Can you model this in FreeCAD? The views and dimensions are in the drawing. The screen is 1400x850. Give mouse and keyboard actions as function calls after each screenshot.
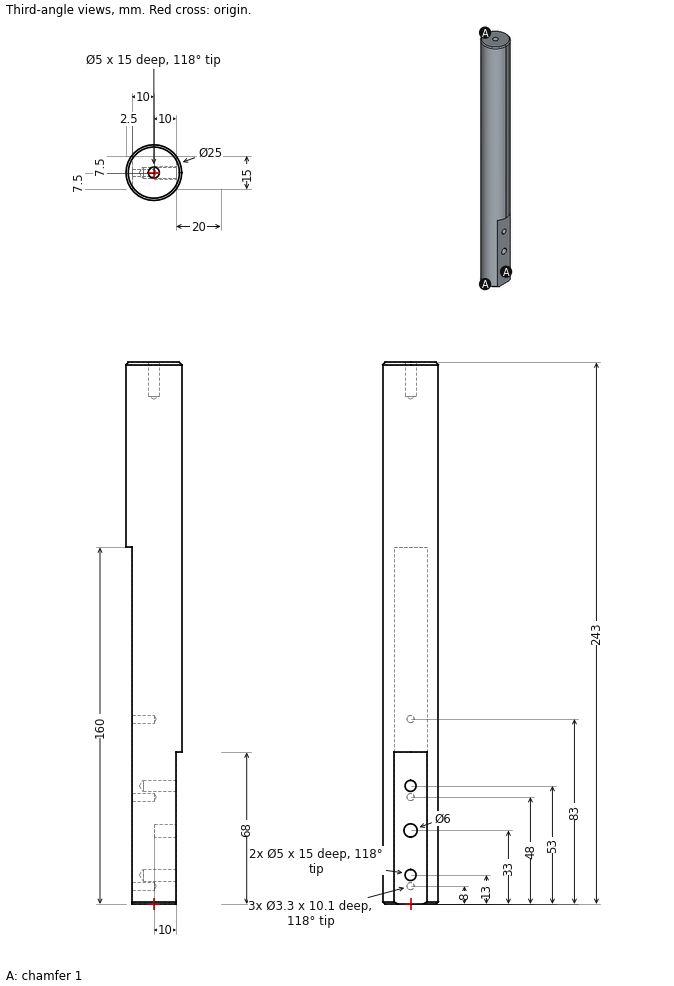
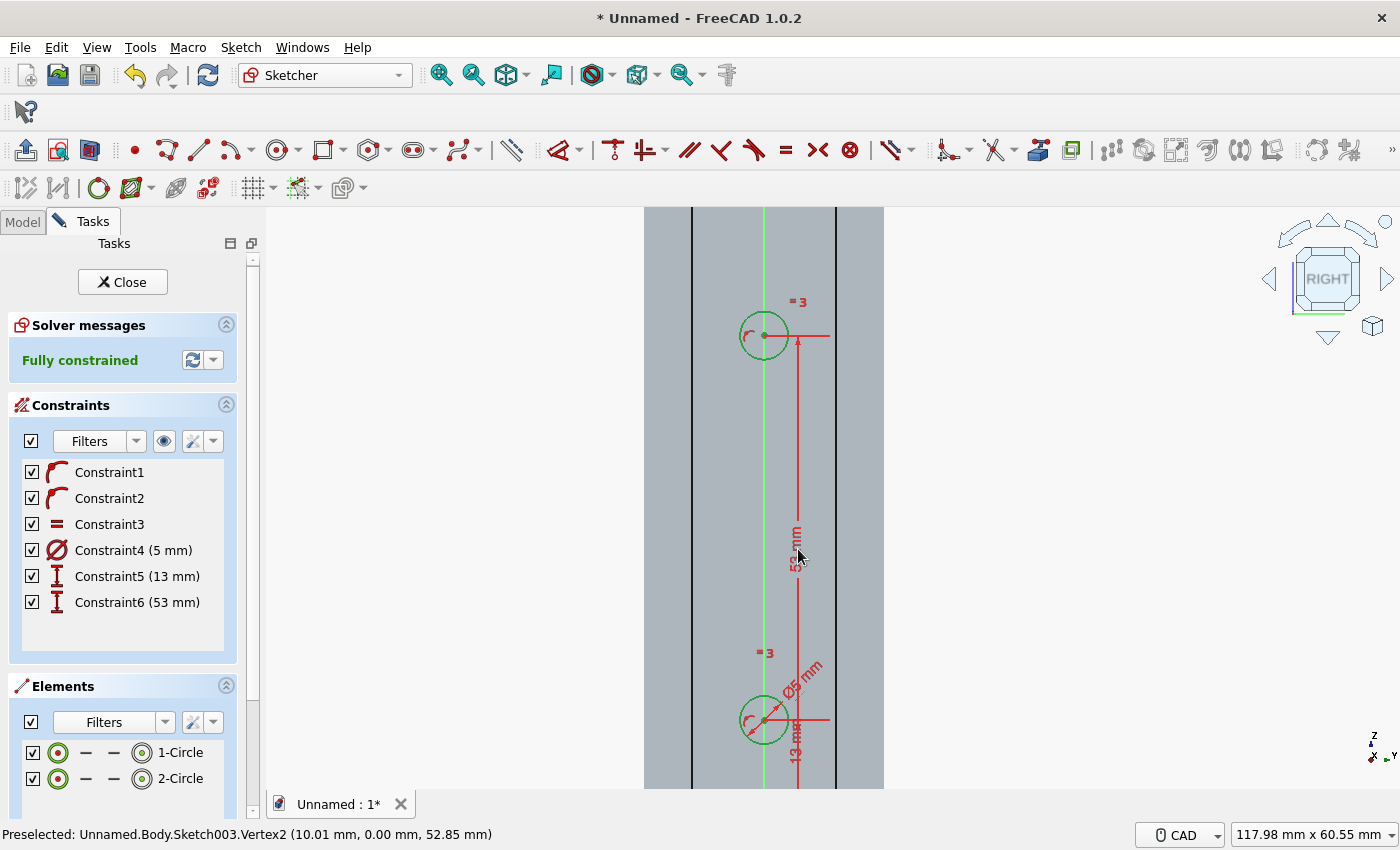
click(123, 282)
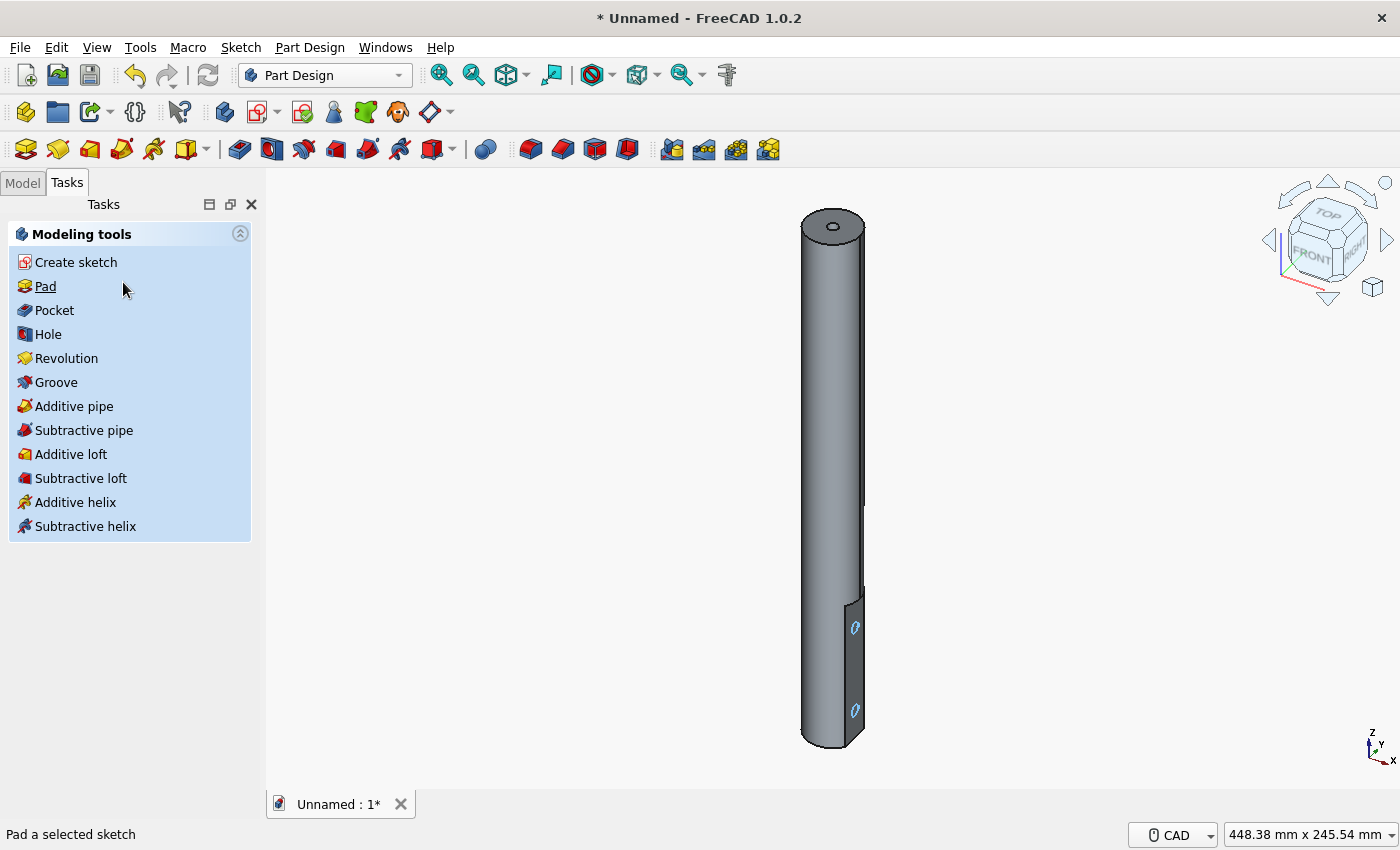
click(272, 150)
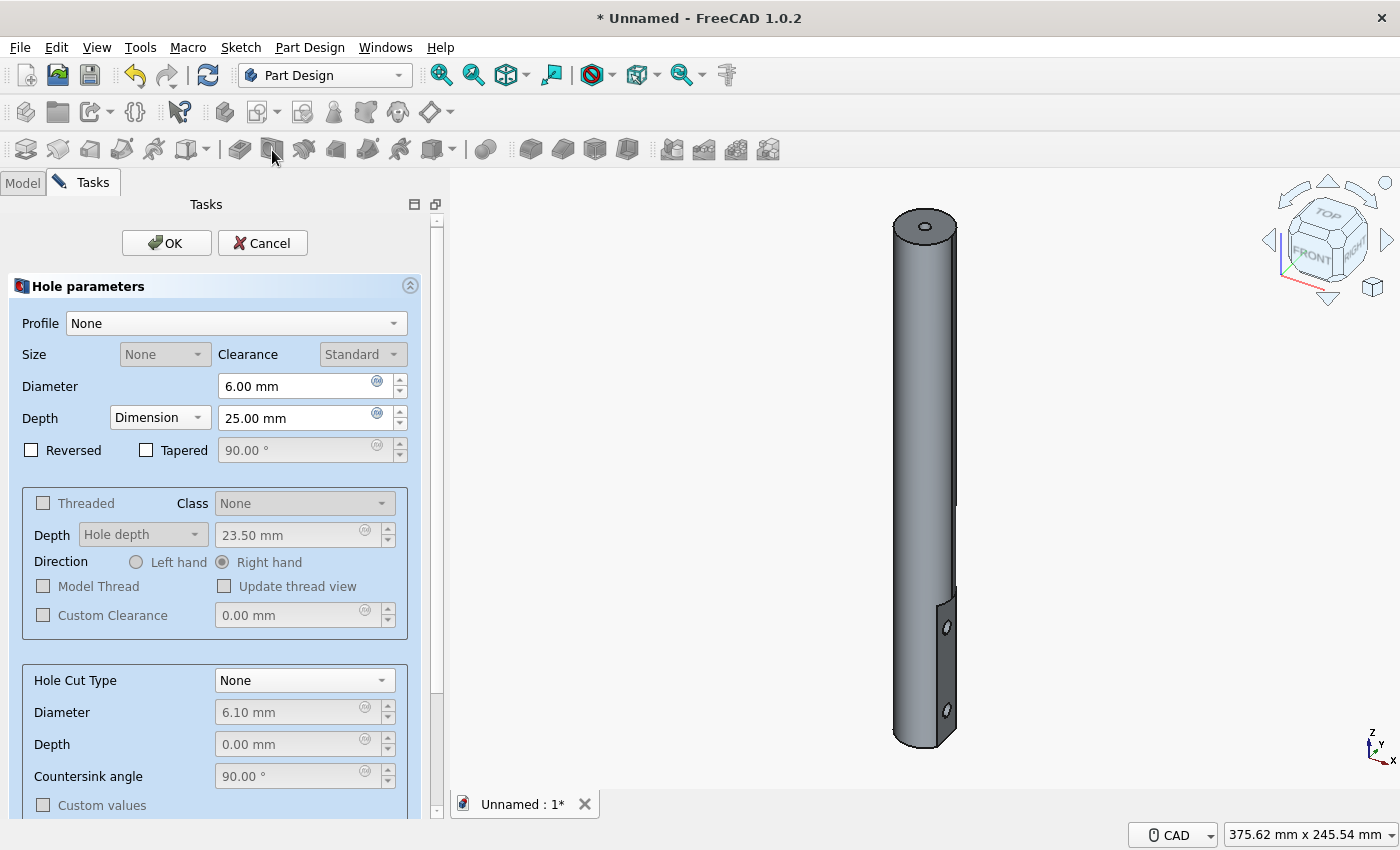
triple_click(305, 386)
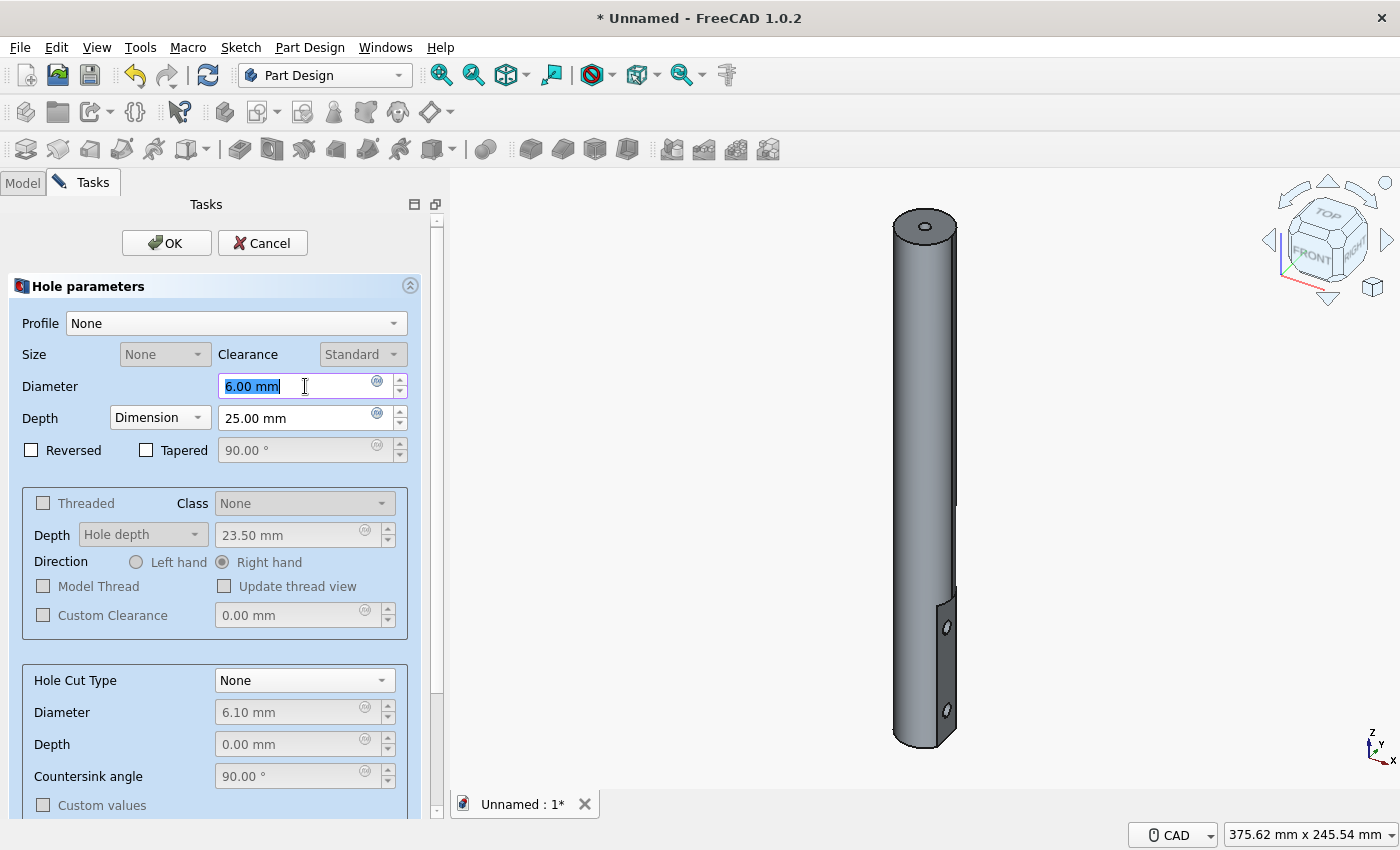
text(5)
key(Tab)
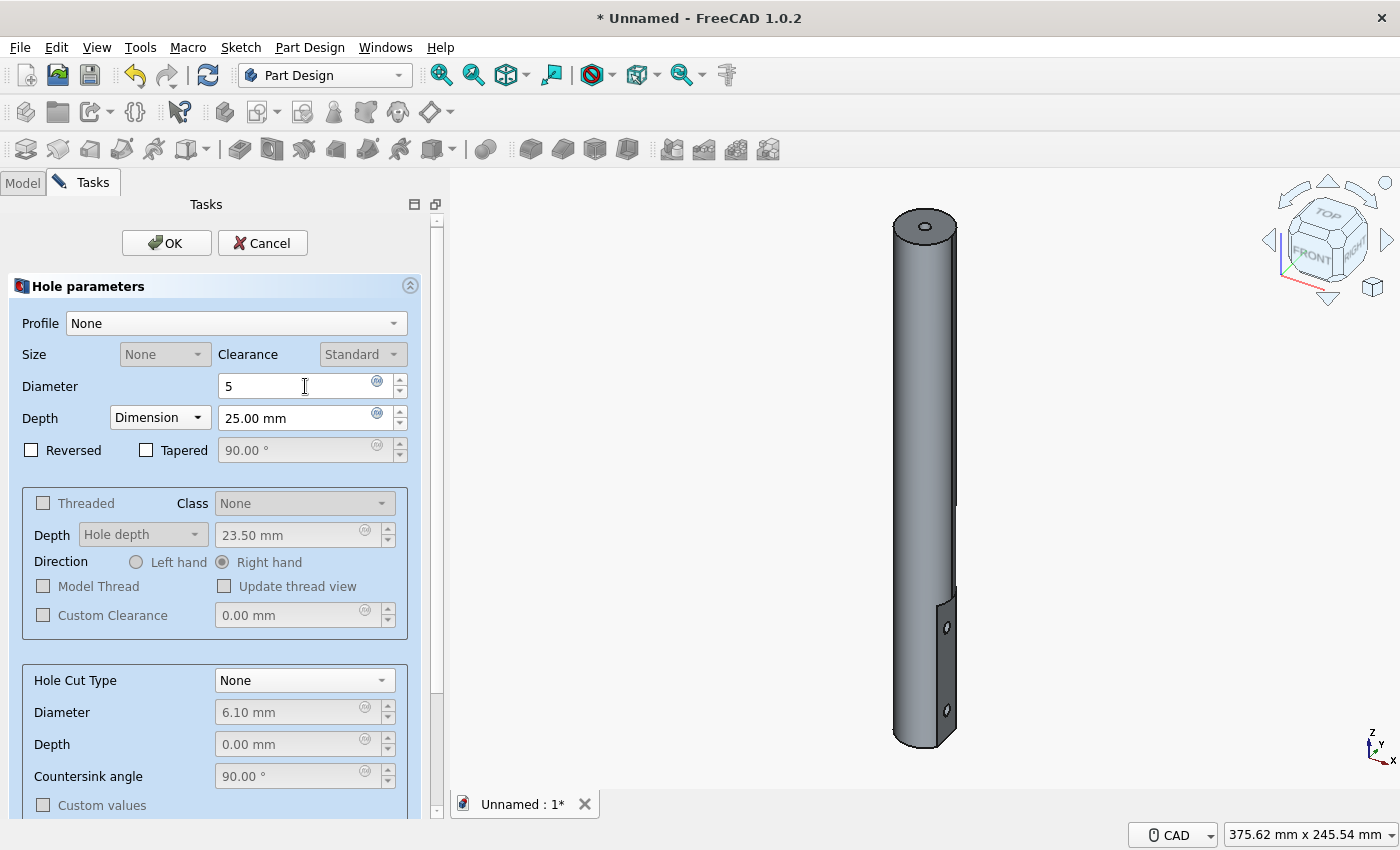
triple_click(305, 418)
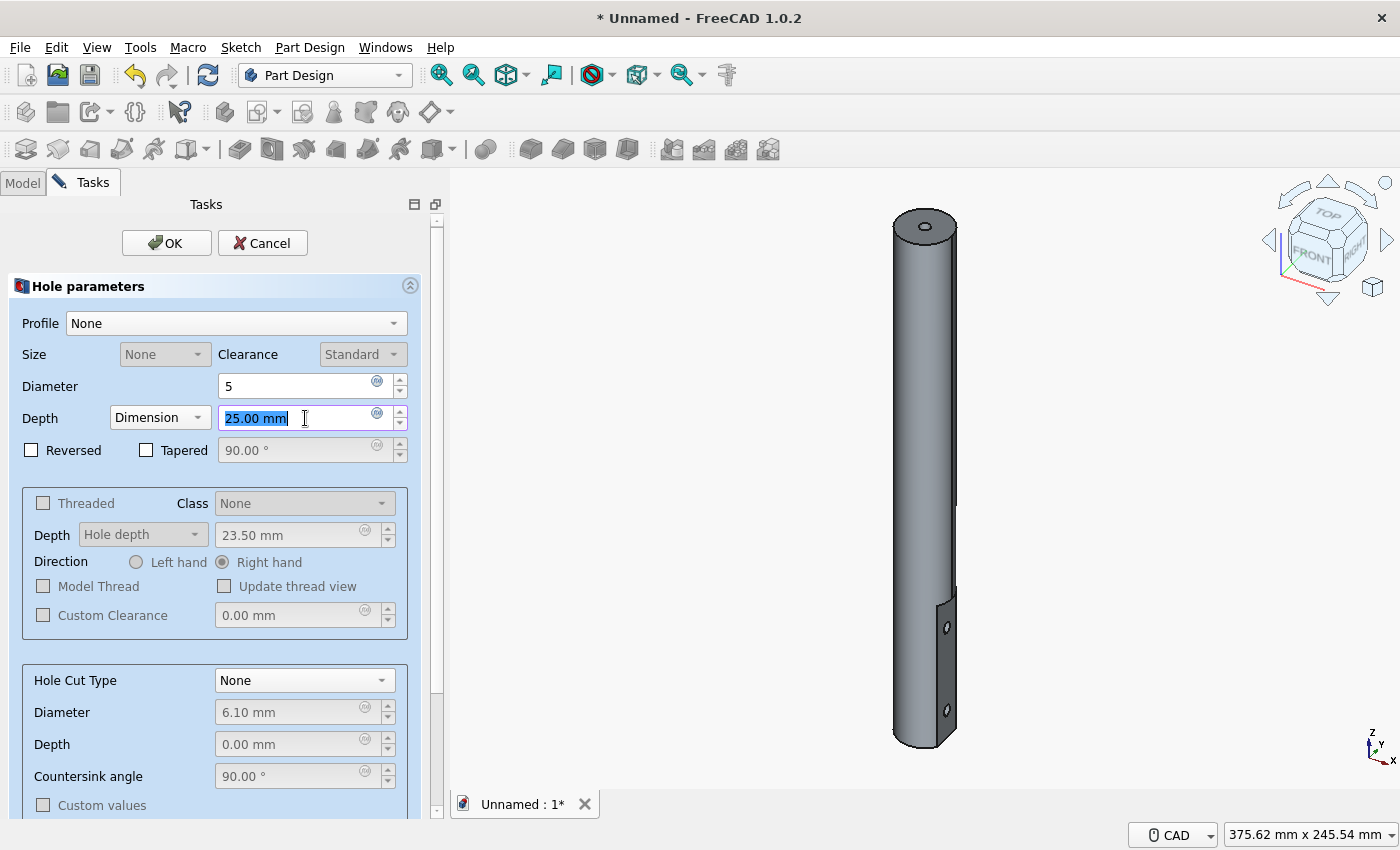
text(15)
key(Tab)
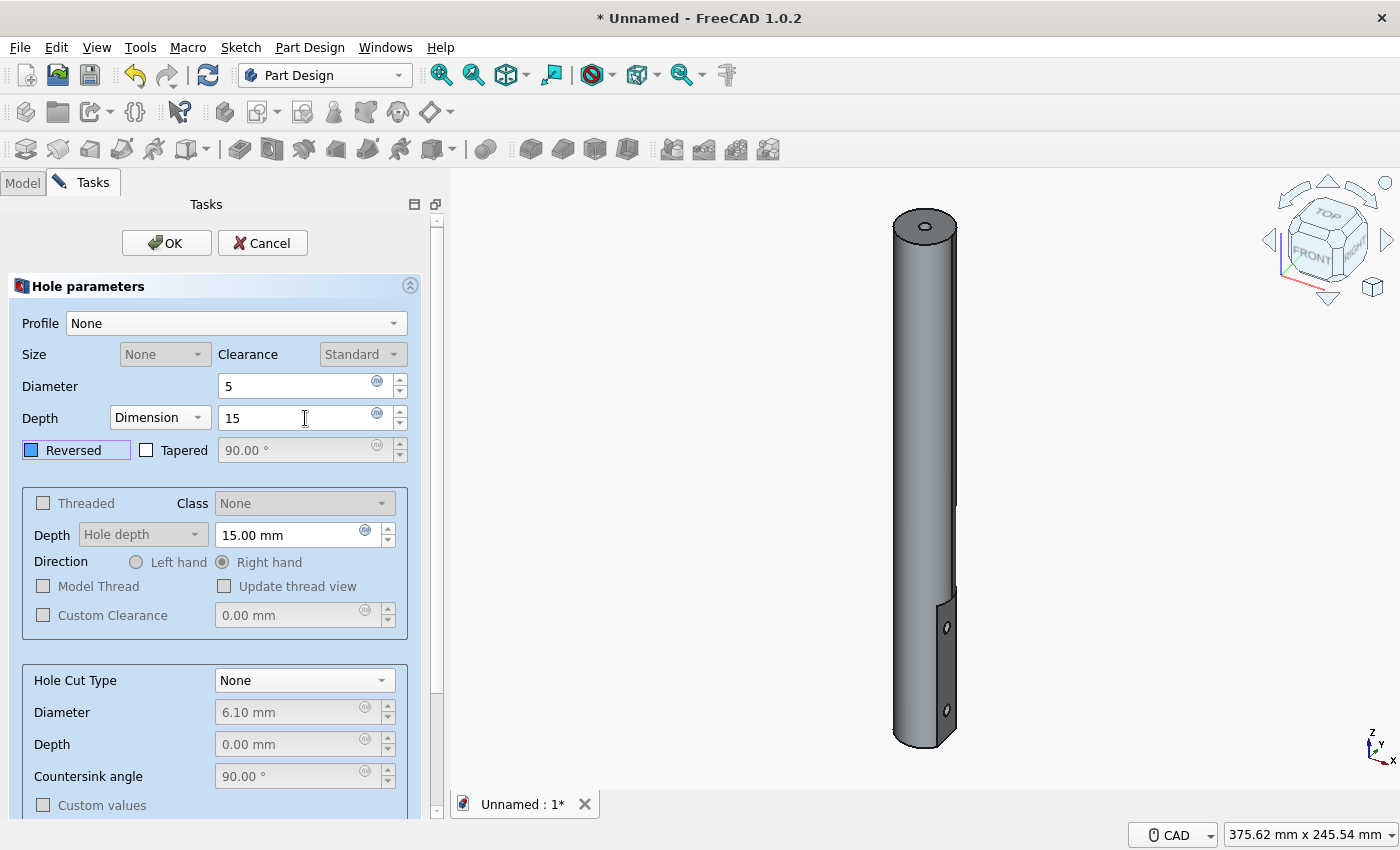
click(167, 243)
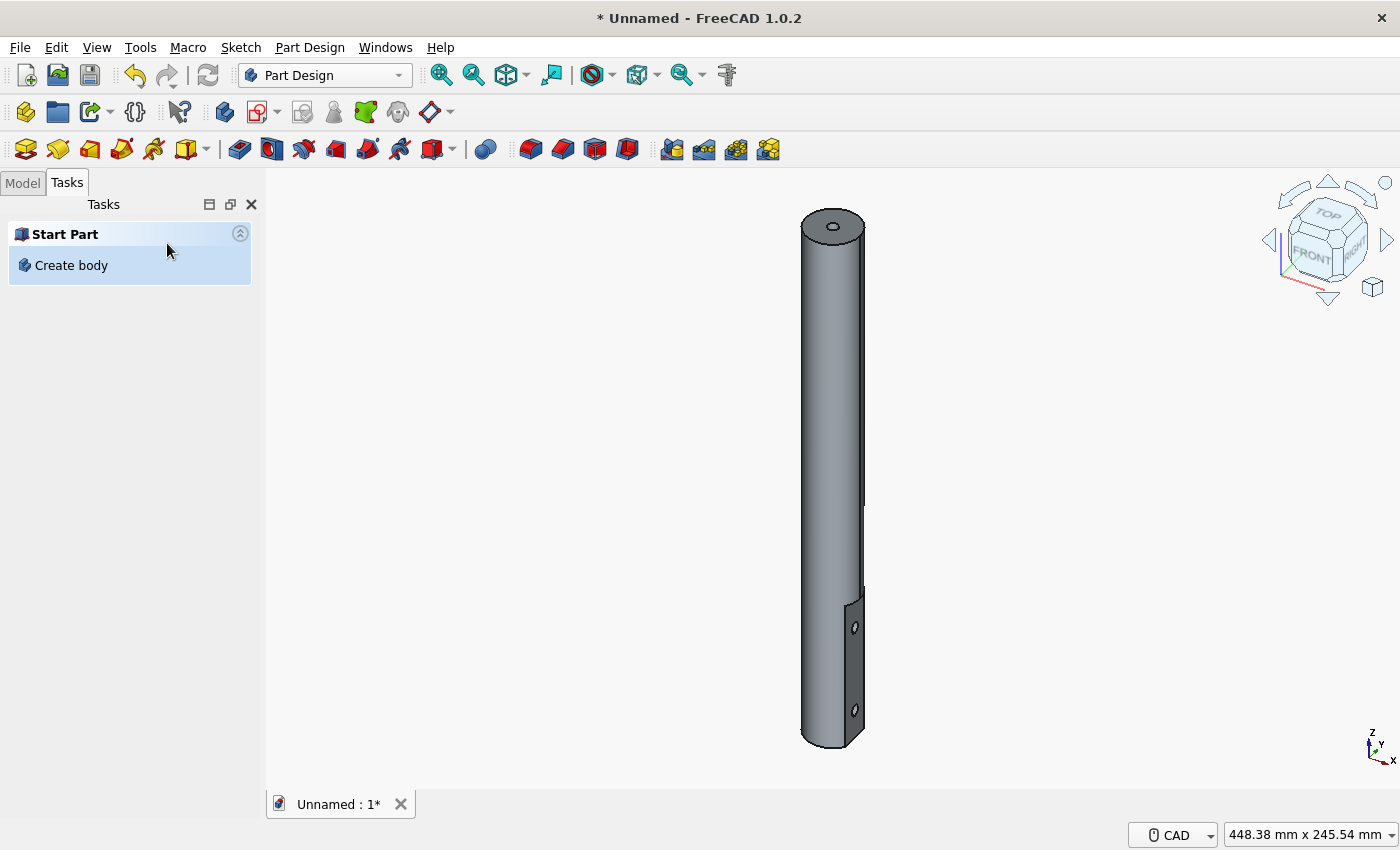
key(5)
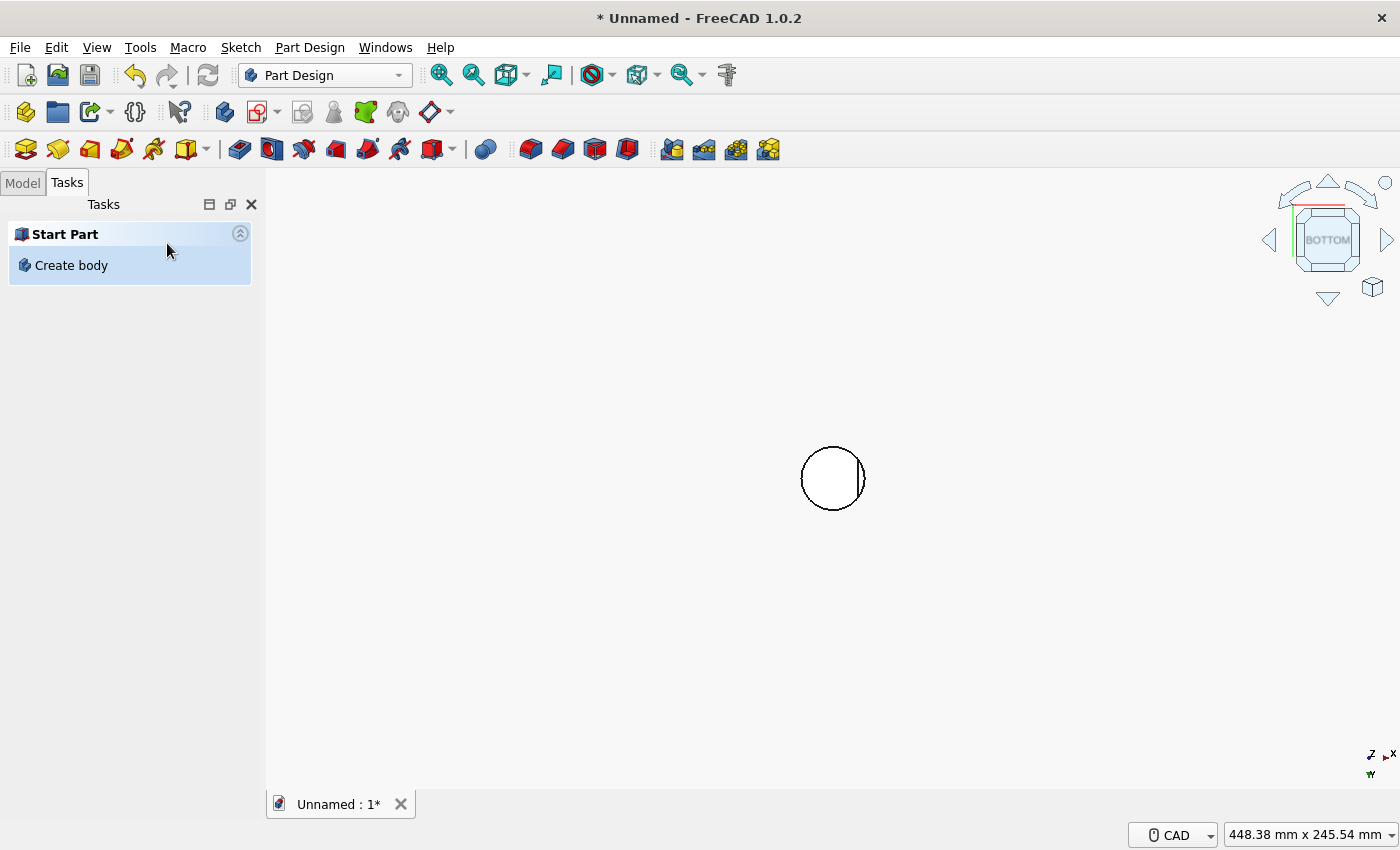
key(v)
key(f)